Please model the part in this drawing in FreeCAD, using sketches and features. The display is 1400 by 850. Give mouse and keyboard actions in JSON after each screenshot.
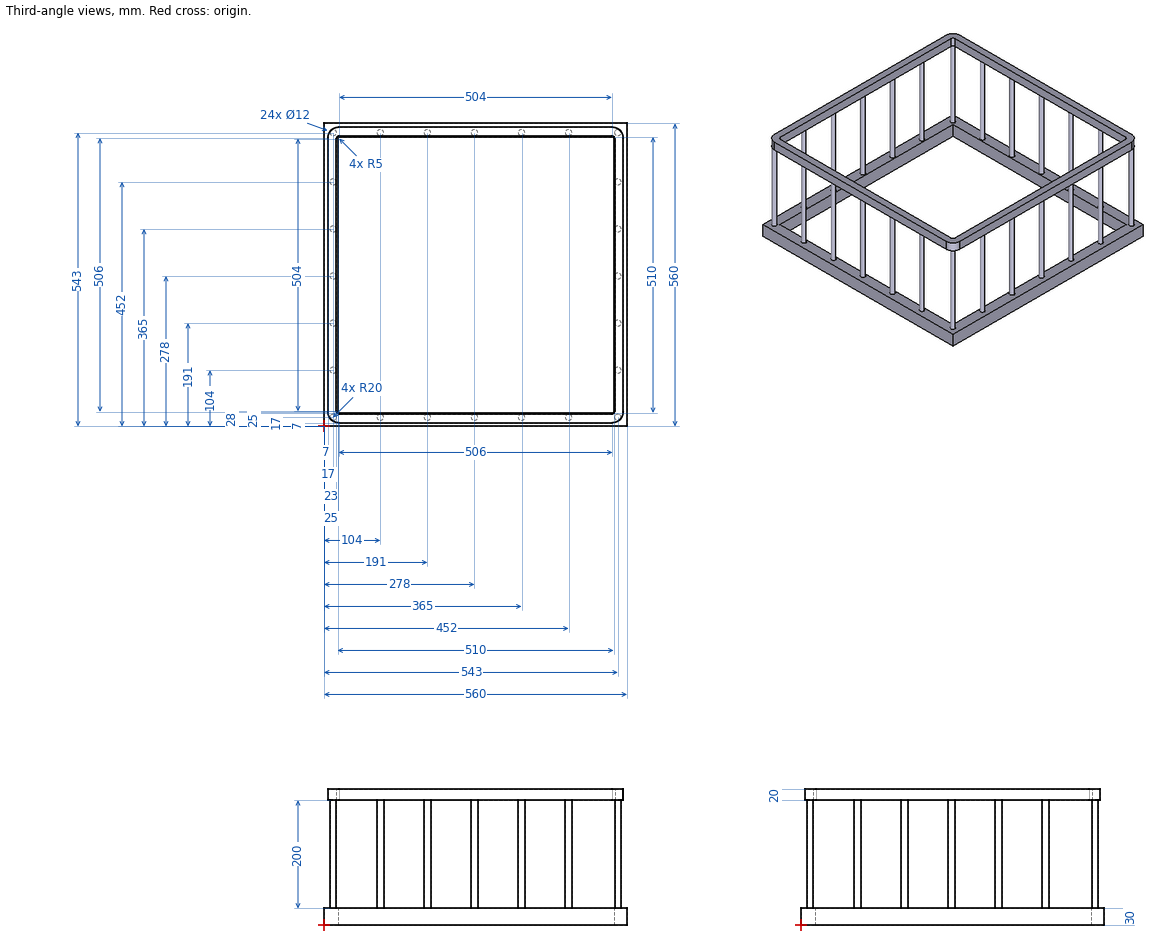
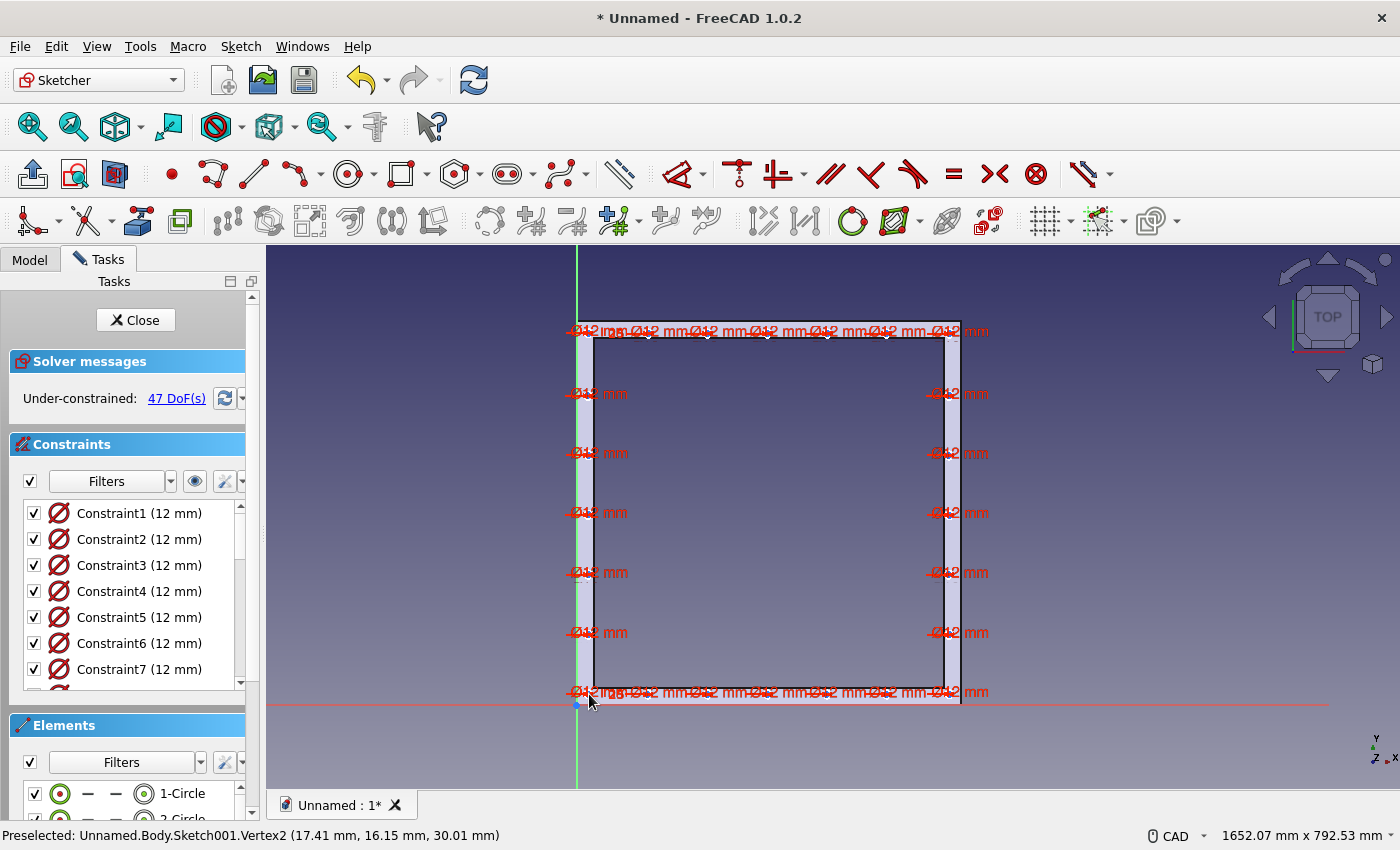
{"action": "left_click", "coordinate": [588, 694]}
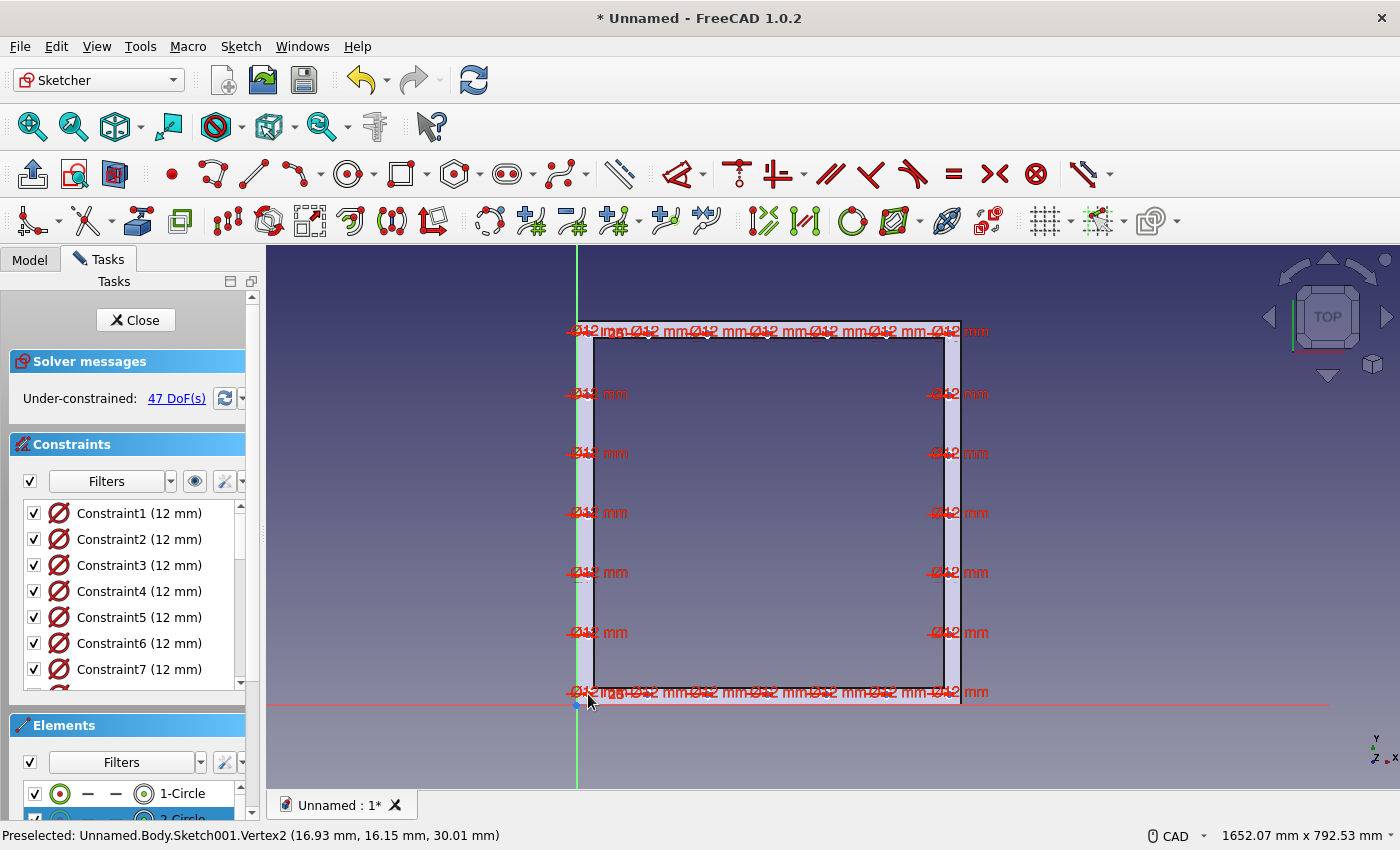
{"action": "left_click", "coordinate": [949, 694]}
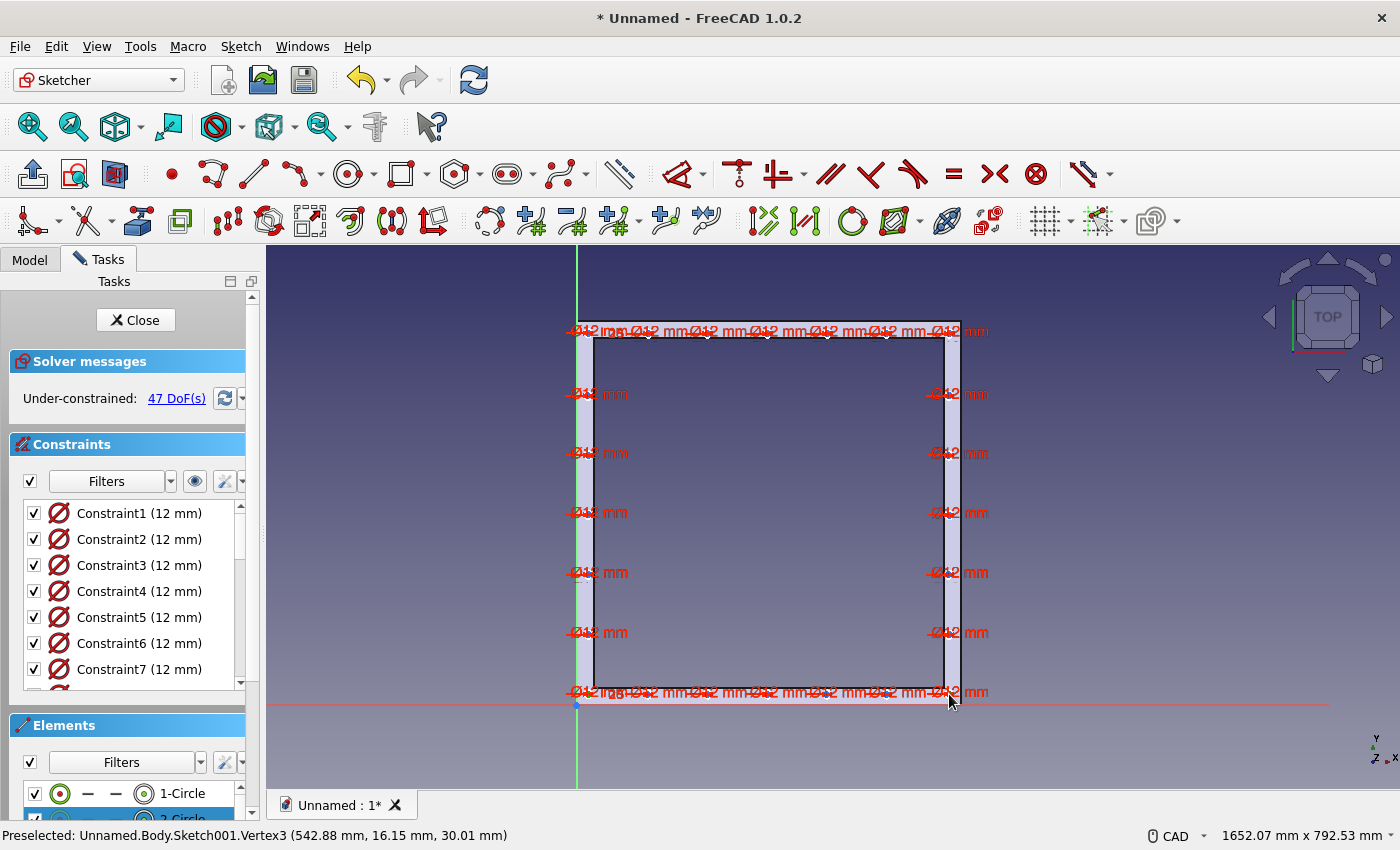
{"action": "left_click", "coordinate": [804, 174]}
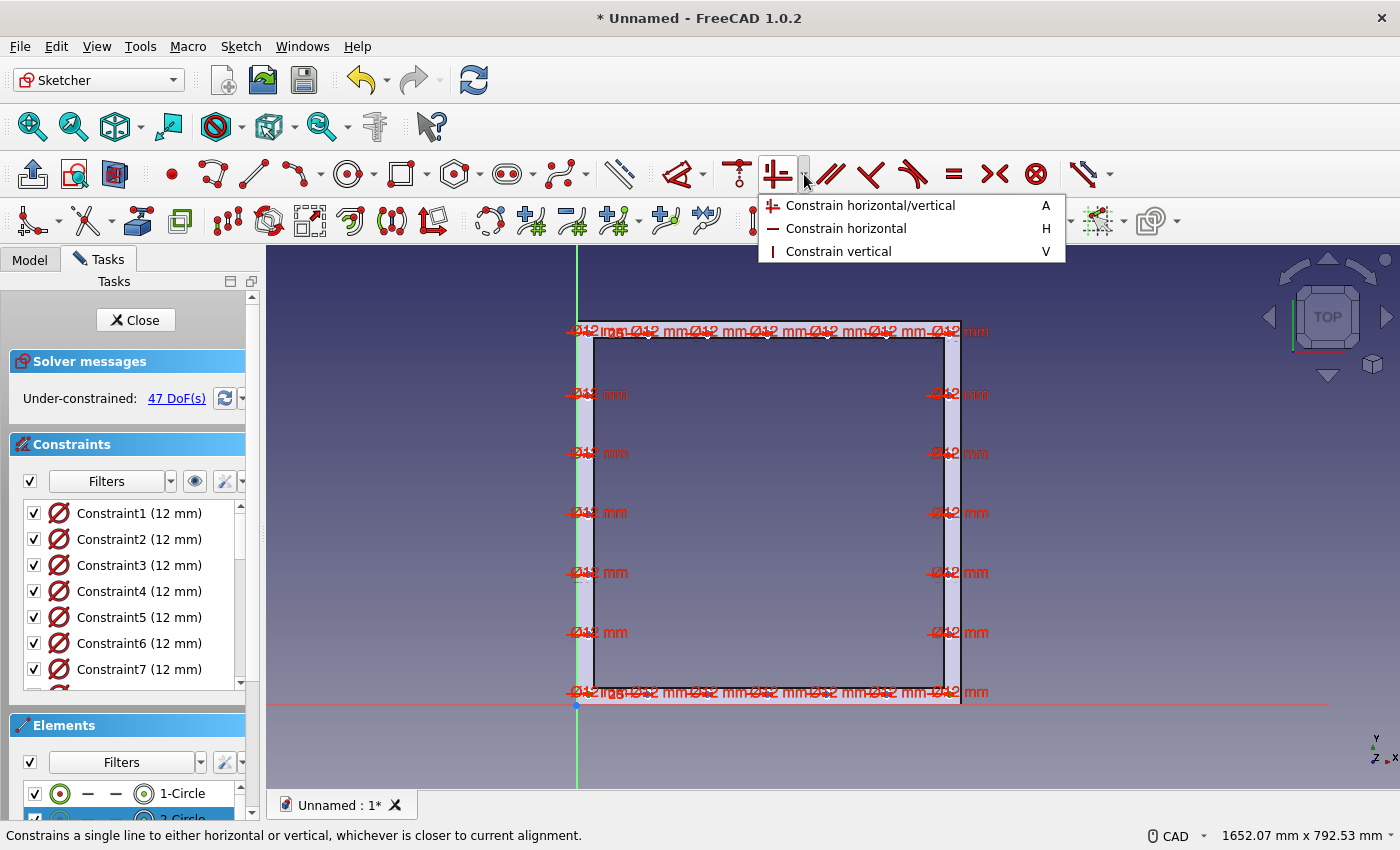
{"action": "left_click", "coordinate": [912, 228]}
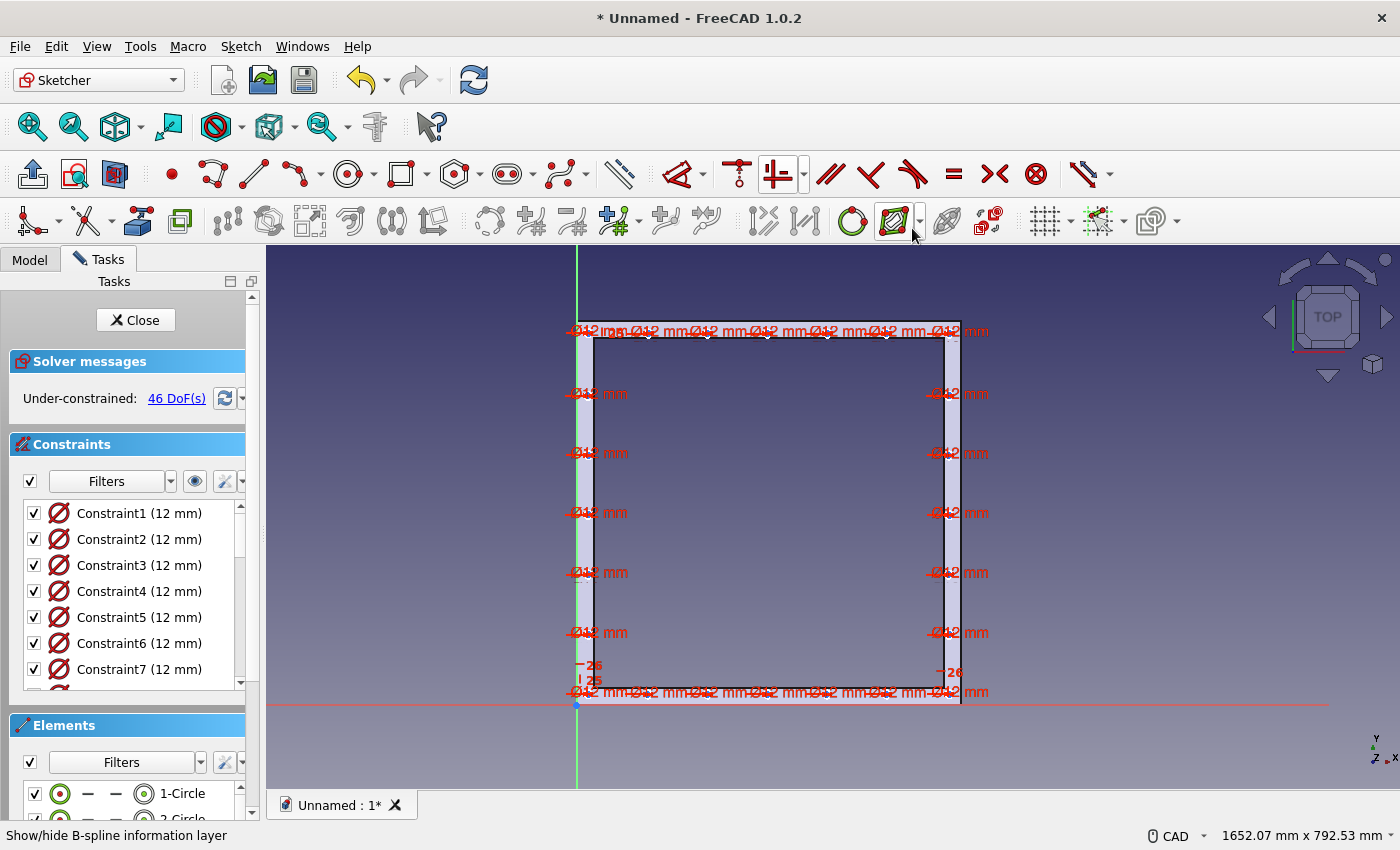
{"action": "left_click", "coordinate": [949, 694]}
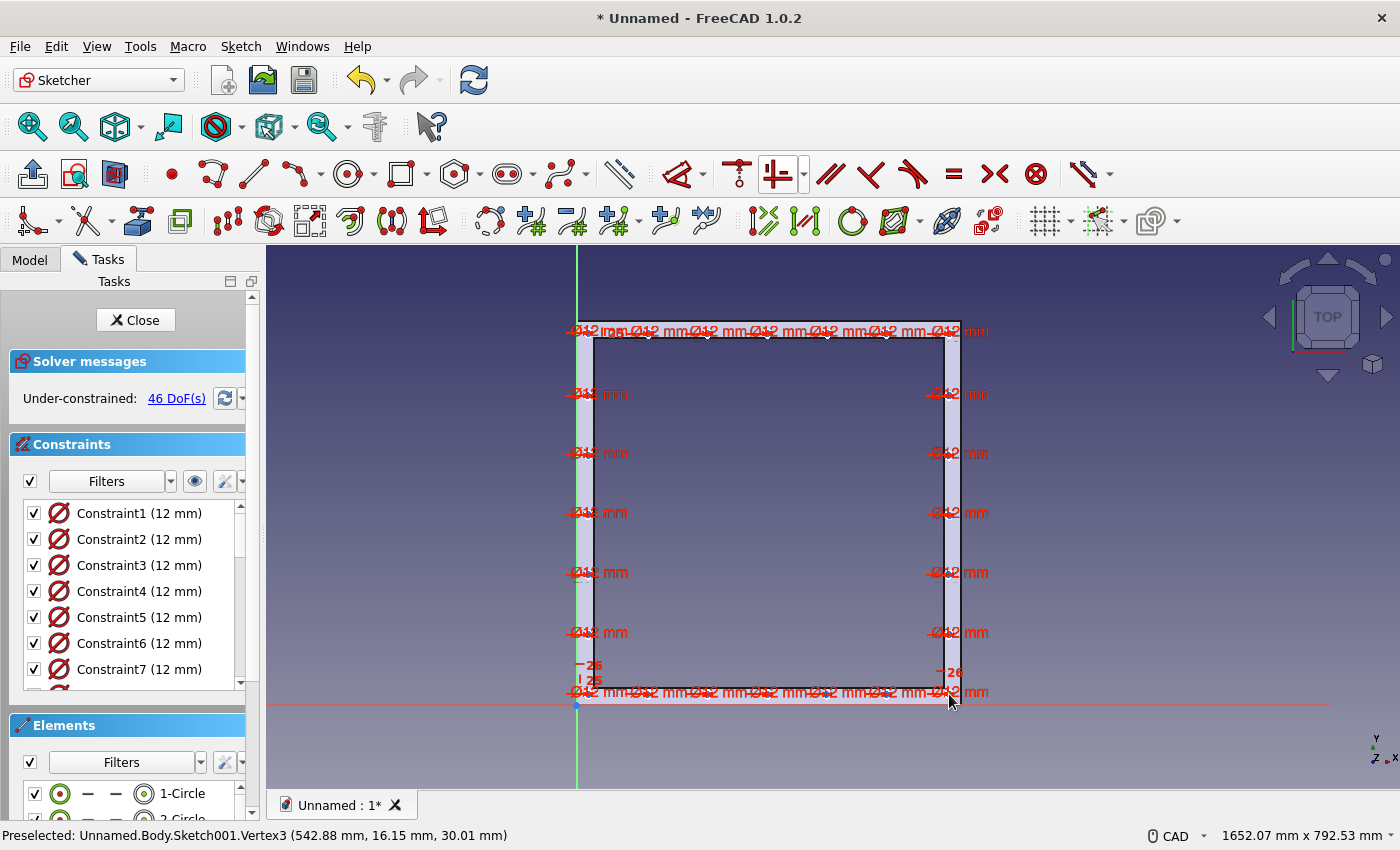
{"action": "left_click", "coordinate": [949, 334]}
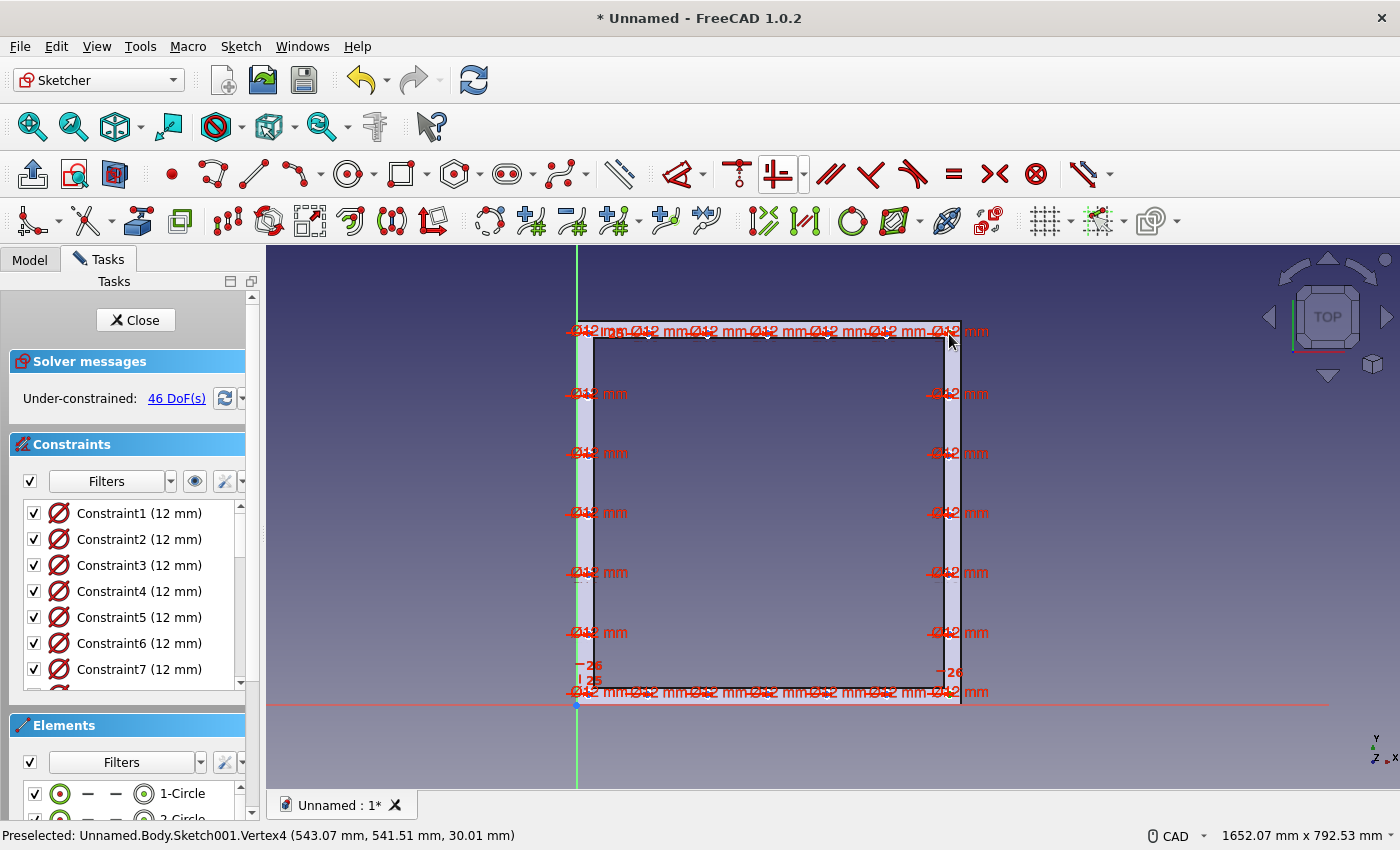
{"action": "key", "text": "v"}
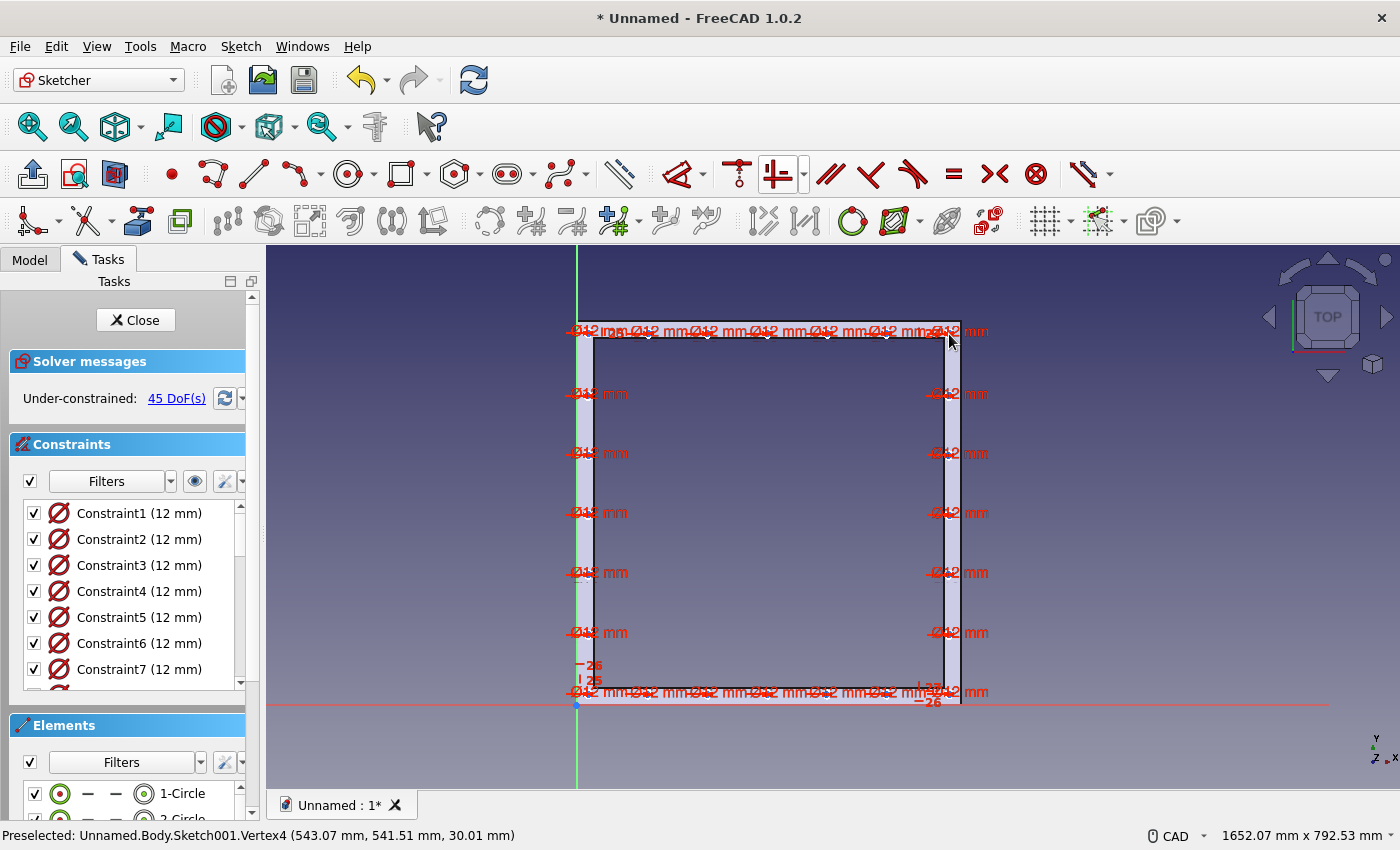
{"action": "left_click", "coordinate": [588, 333]}